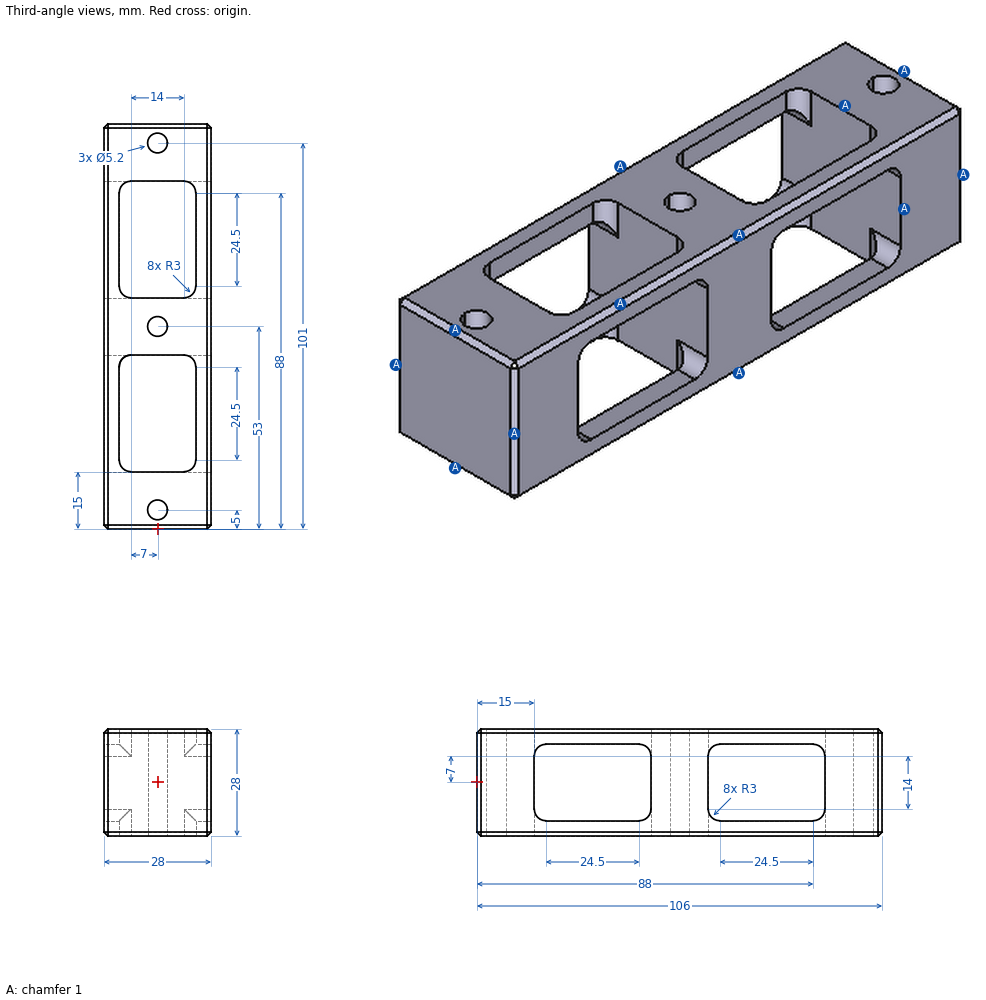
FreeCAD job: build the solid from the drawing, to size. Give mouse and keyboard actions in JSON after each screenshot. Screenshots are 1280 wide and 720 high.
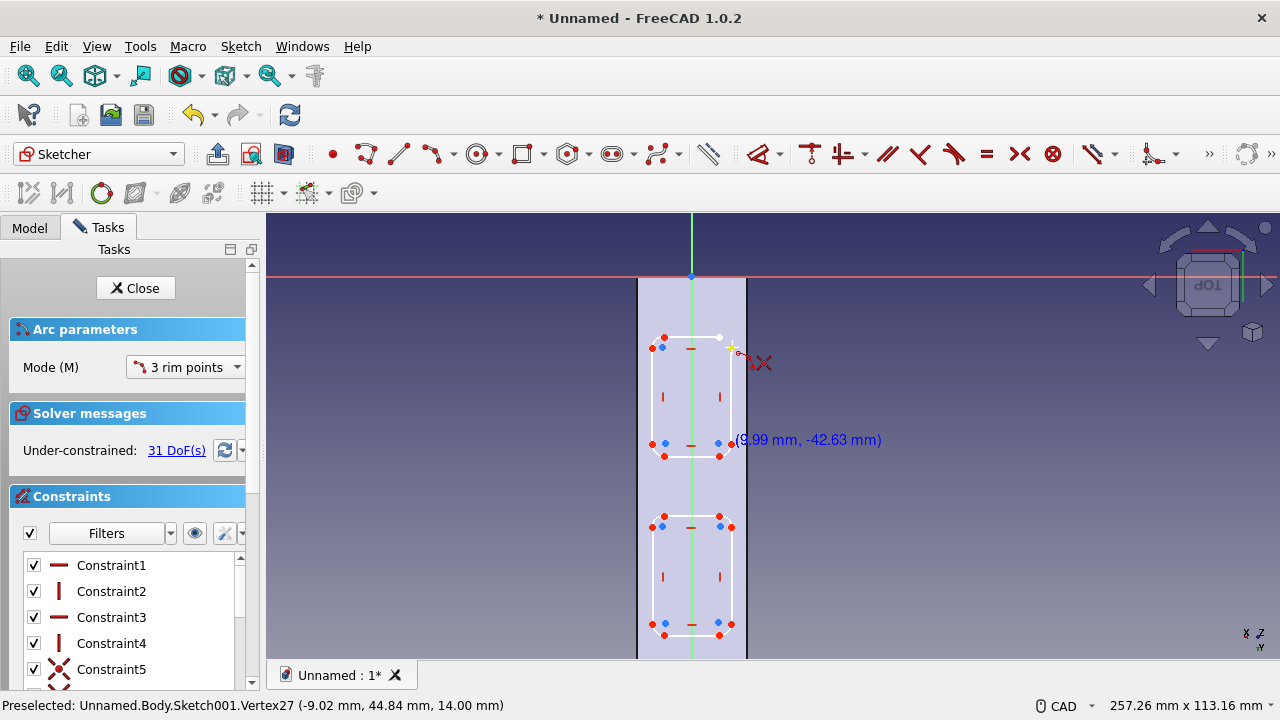
{"action": "left_click", "coordinate": [731, 349]}
{"action": "left_click", "coordinate": [719, 337]}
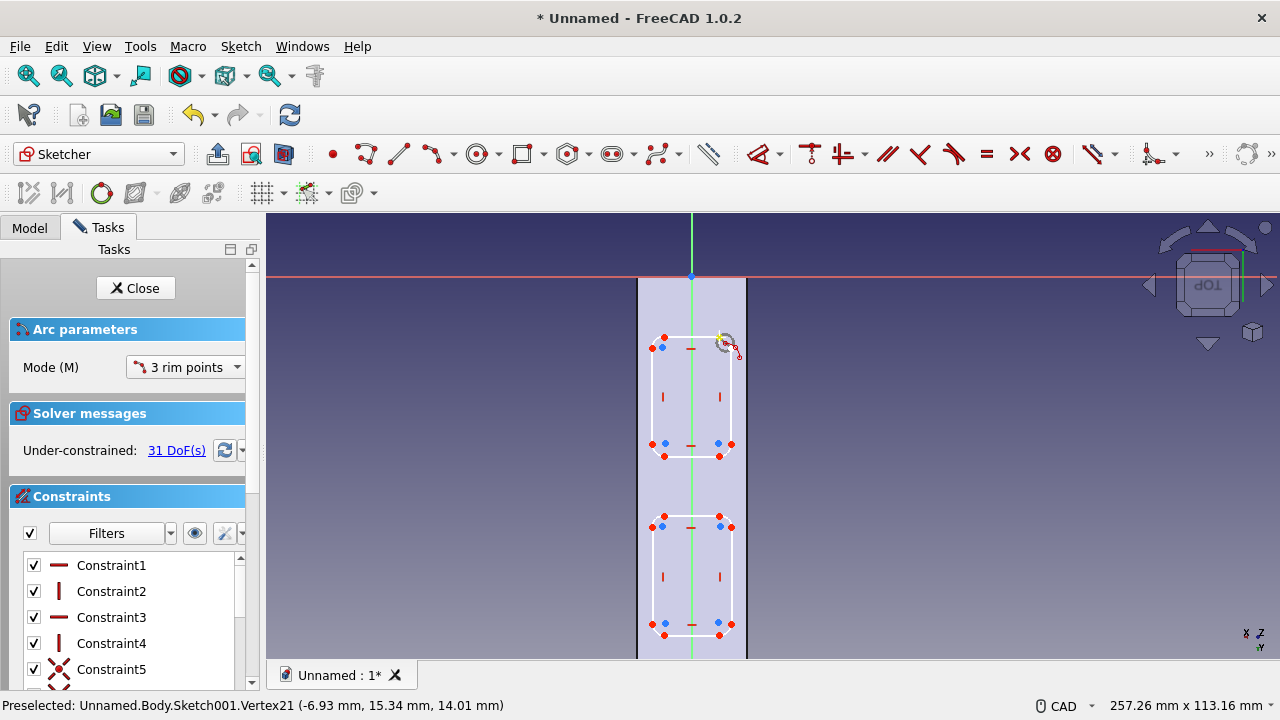
{"action": "scroll", "coordinate": [728, 339], "scroll_direction": "up", "scroll_amount": 8}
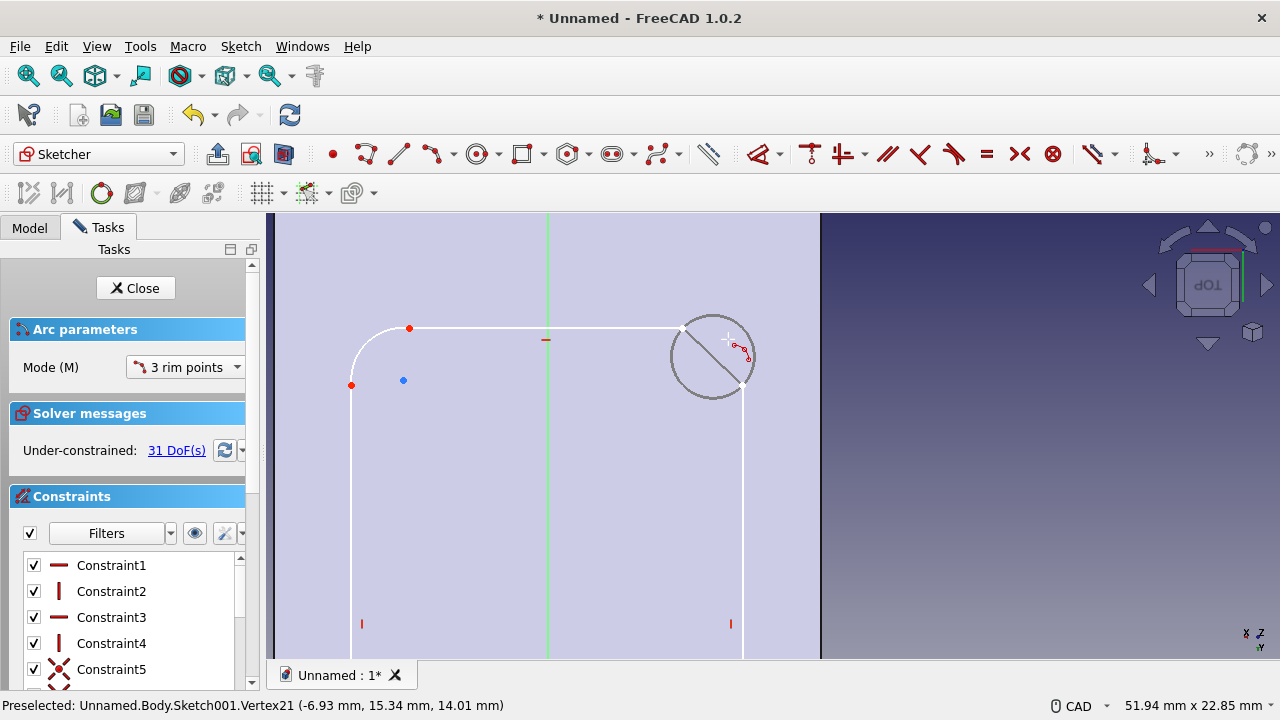
{"action": "left_click", "coordinate": [726, 339]}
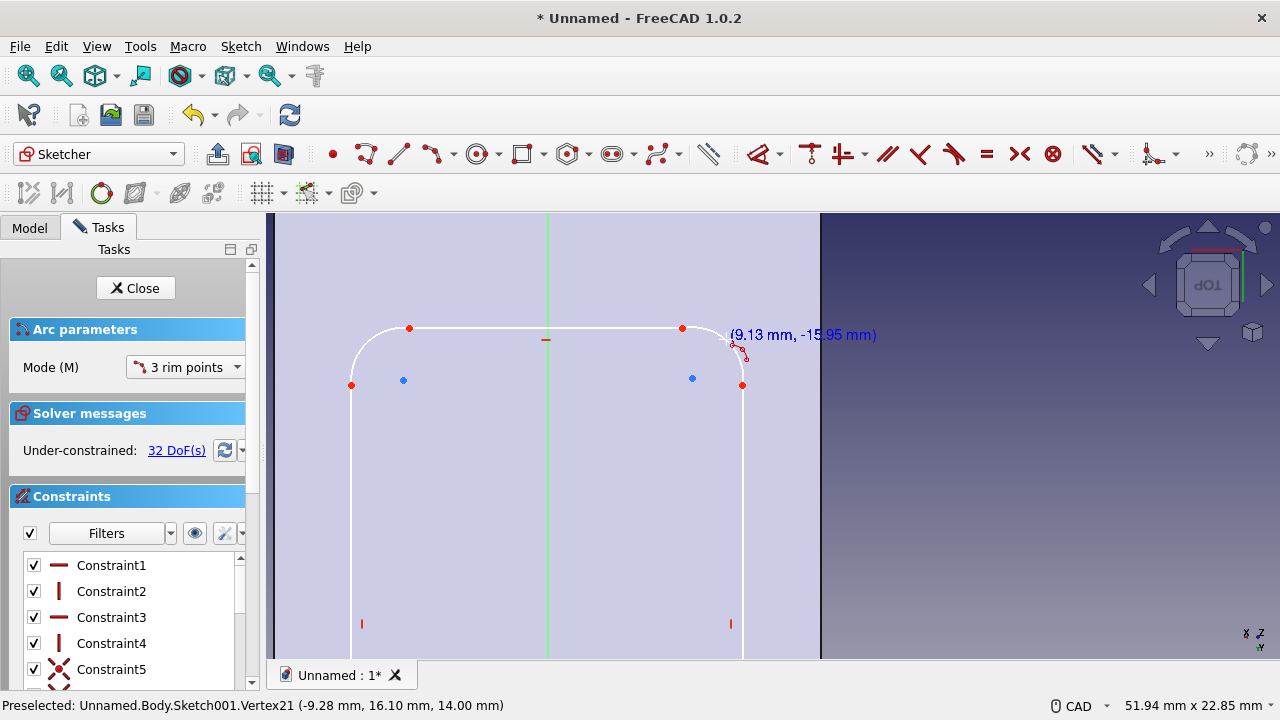
{"action": "left_click", "coordinate": [476, 154]}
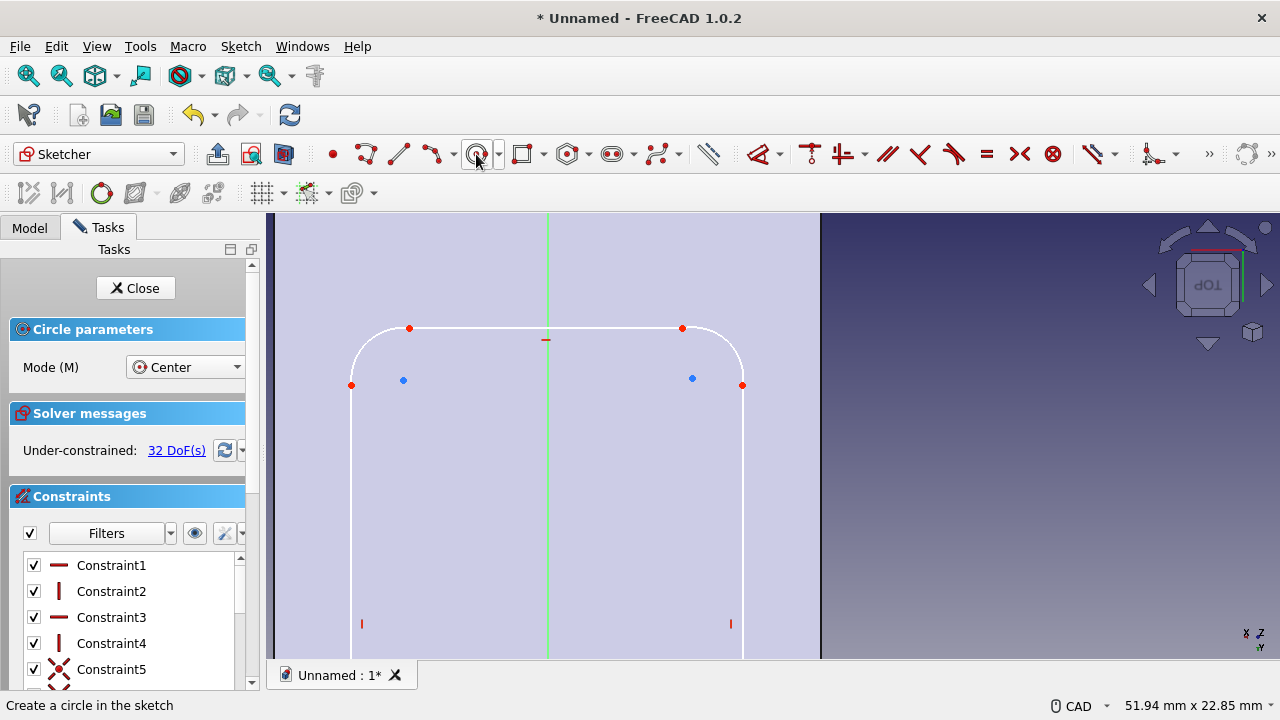
{"action": "scroll", "coordinate": [729, 341], "scroll_direction": "down", "scroll_amount": 10}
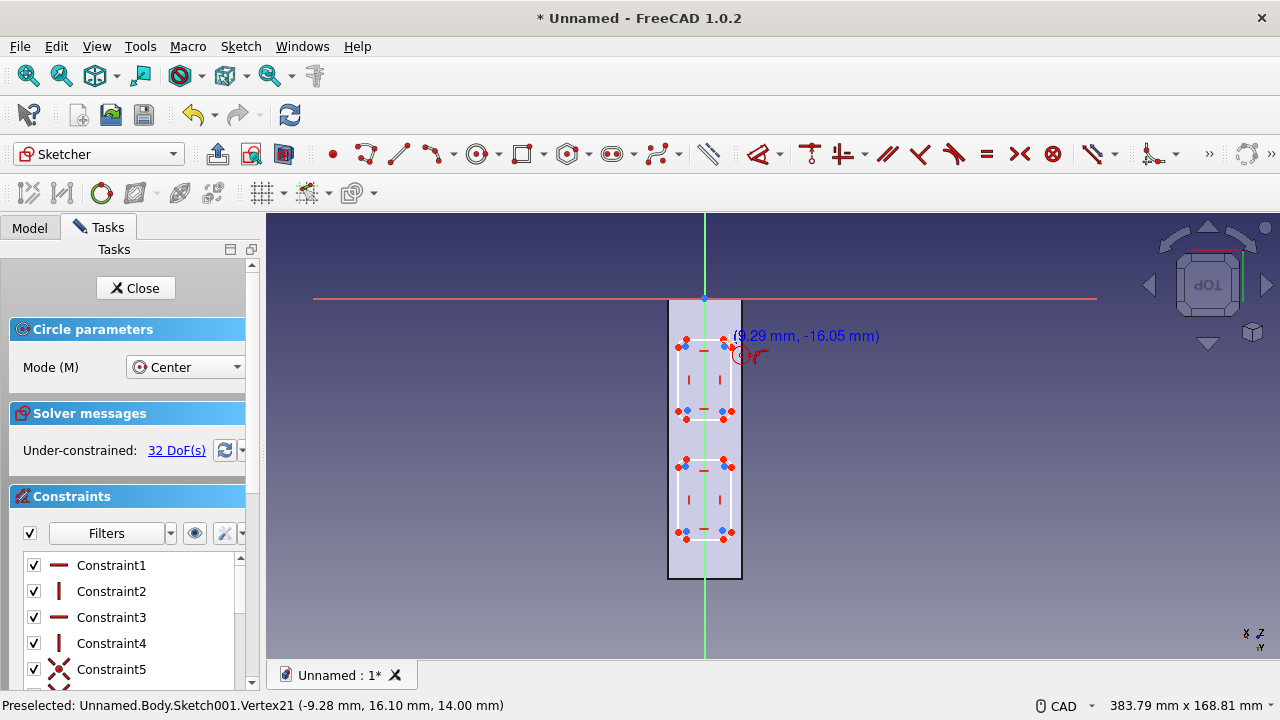
{"action": "scroll", "coordinate": [705, 566], "scroll_direction": "up", "scroll_amount": 6}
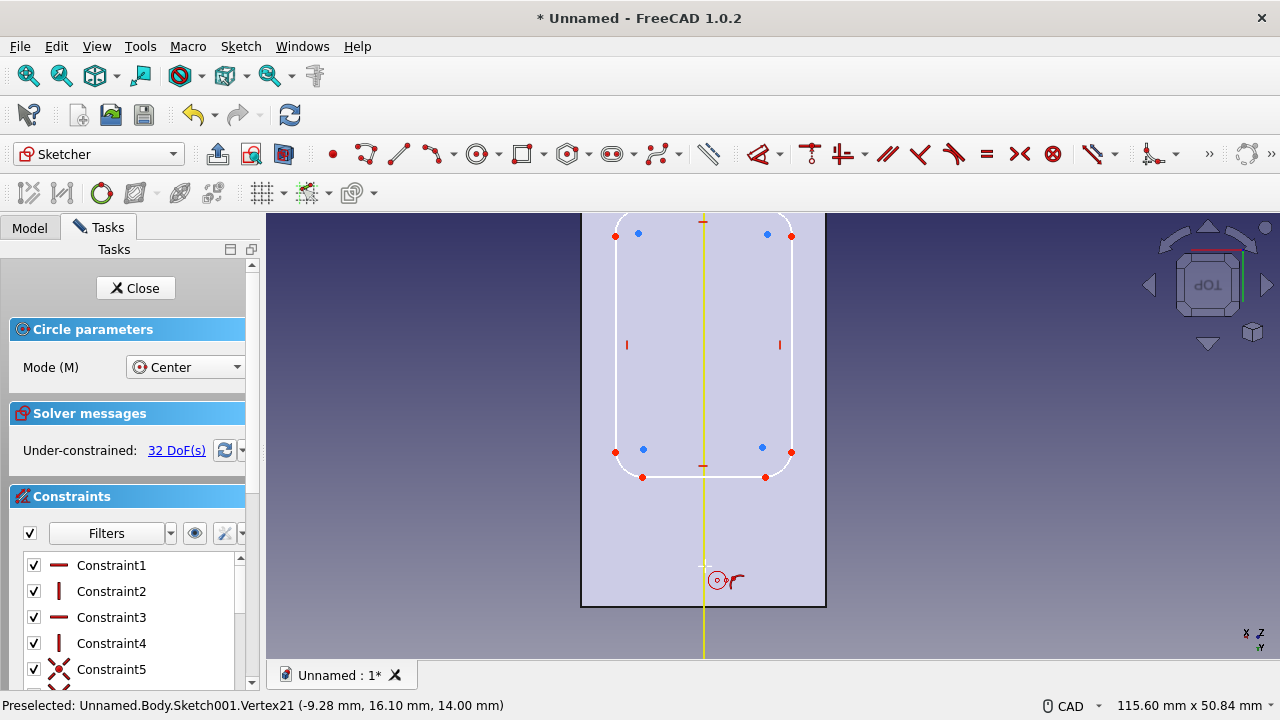
{"action": "left_click", "coordinate": [704, 564]}
{"action": "mouse_move", "coordinate": [720, 547]}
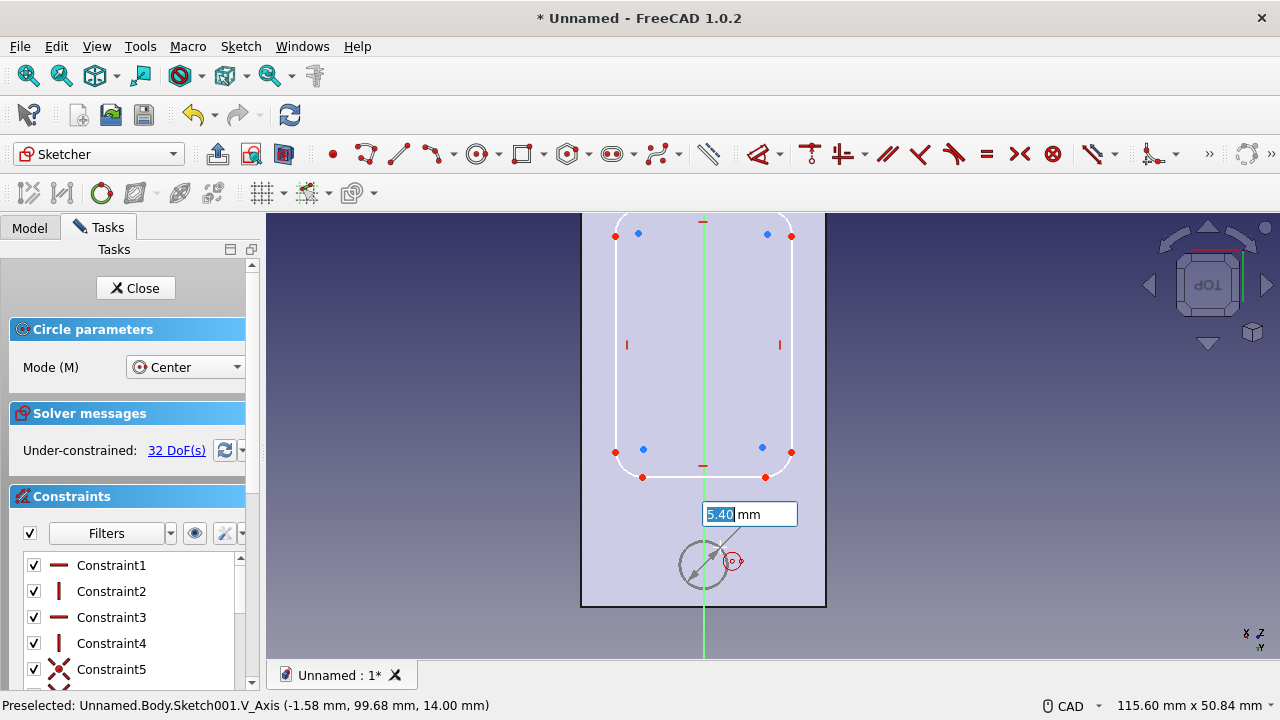
{"action": "type", "text": "5.2"}
{"action": "key", "text": "Return"}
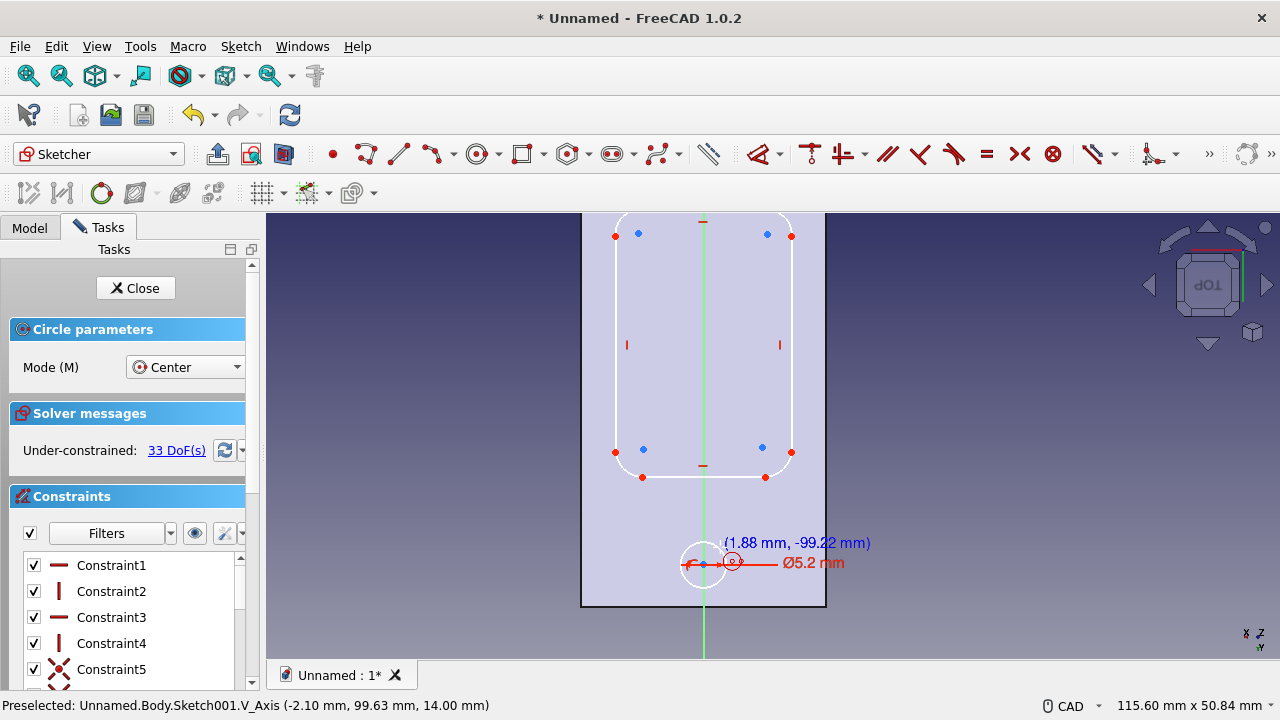
{"action": "scroll", "coordinate": [705, 567], "scroll_direction": "down", "scroll_amount": 6}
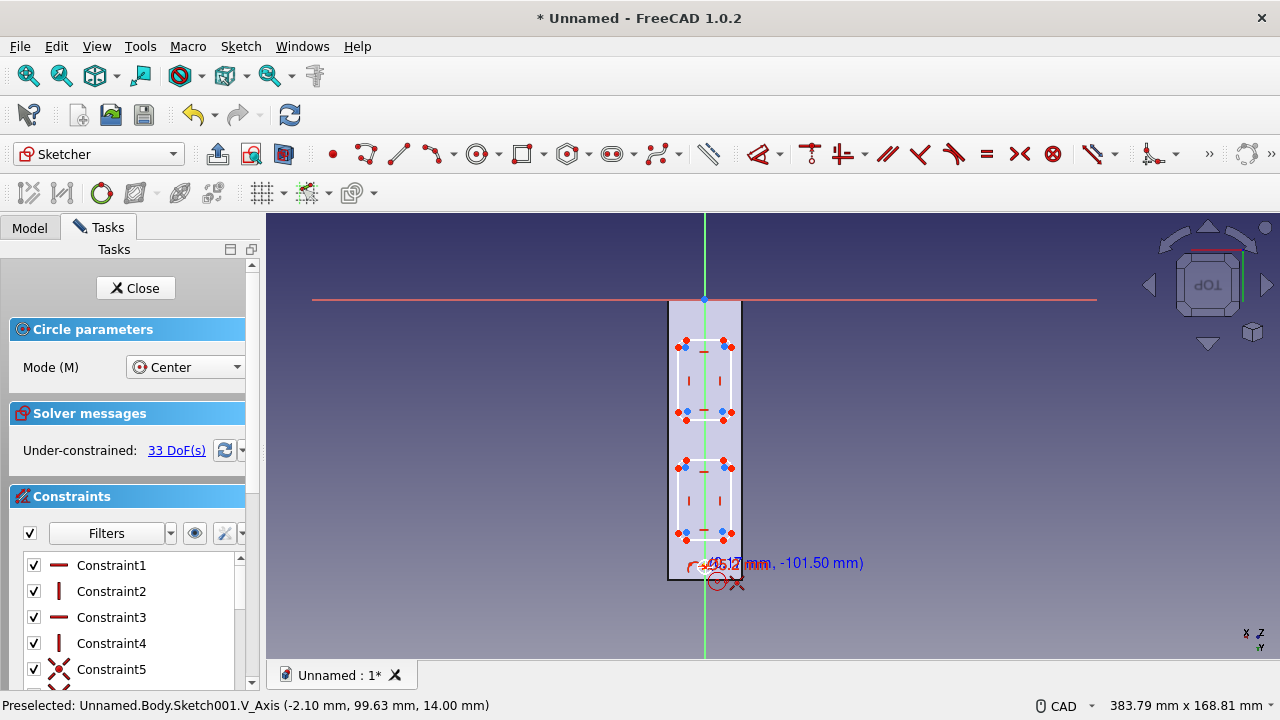
{"action": "scroll", "coordinate": [705, 440], "scroll_direction": "up", "scroll_amount": 6}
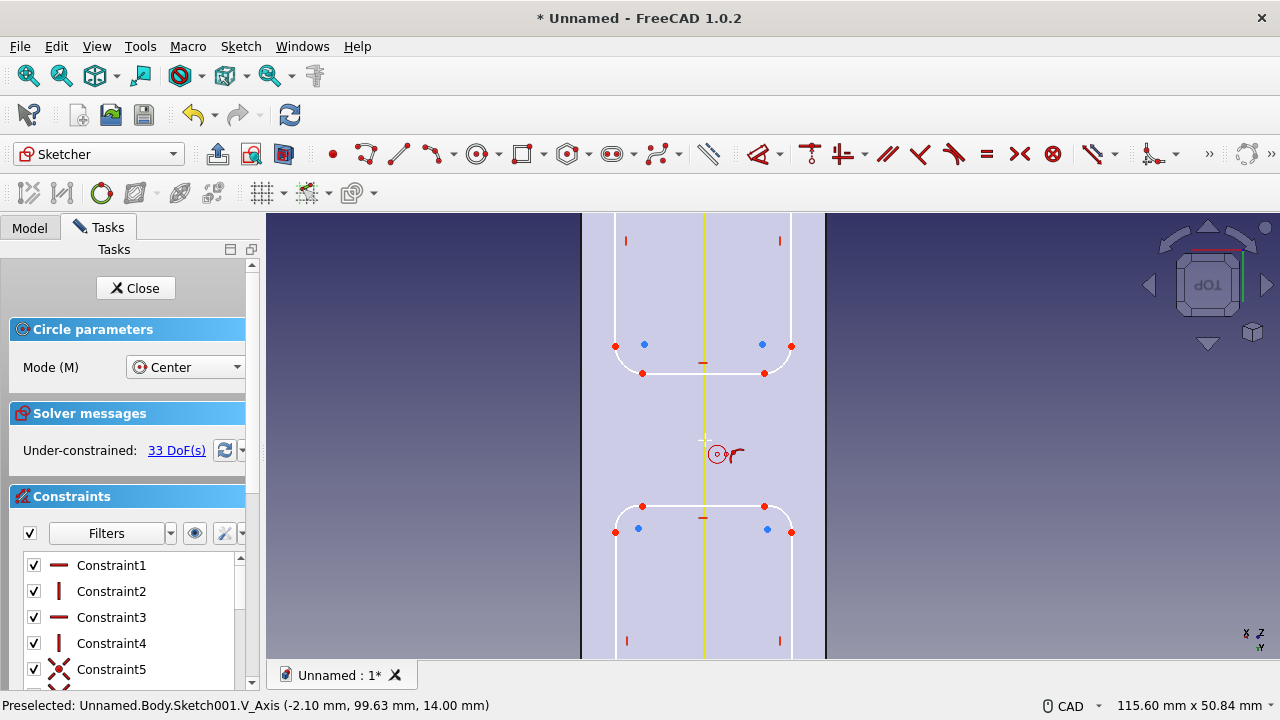
{"action": "left_click", "coordinate": [704, 438]}
{"action": "mouse_move", "coordinate": [720, 422]}